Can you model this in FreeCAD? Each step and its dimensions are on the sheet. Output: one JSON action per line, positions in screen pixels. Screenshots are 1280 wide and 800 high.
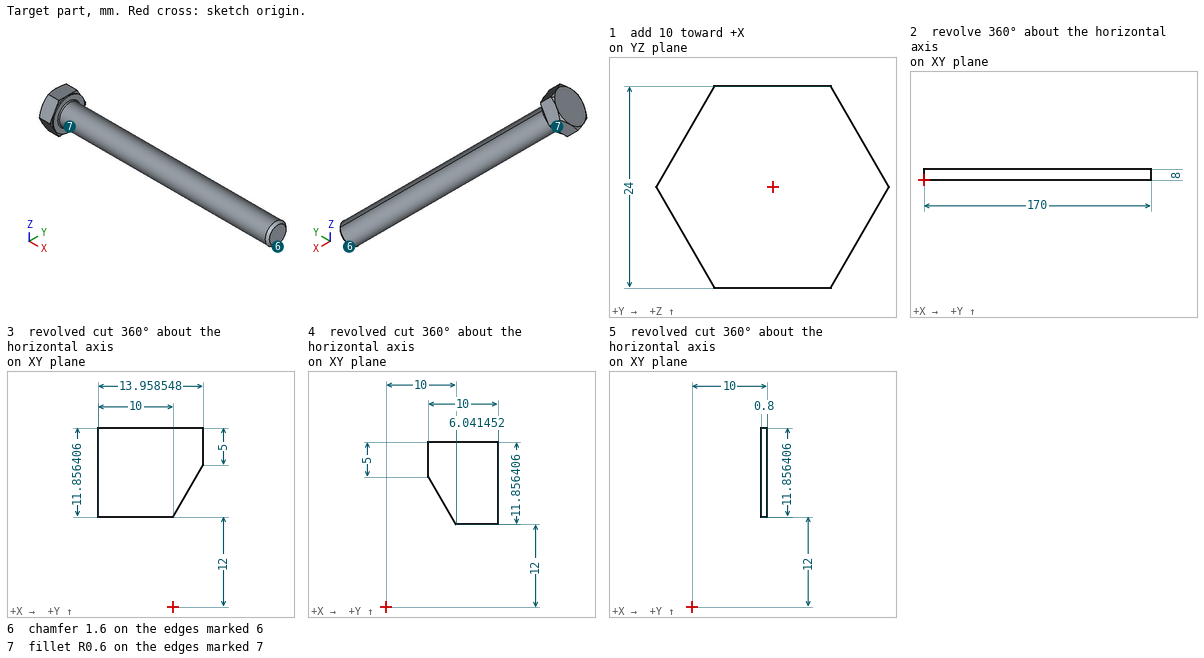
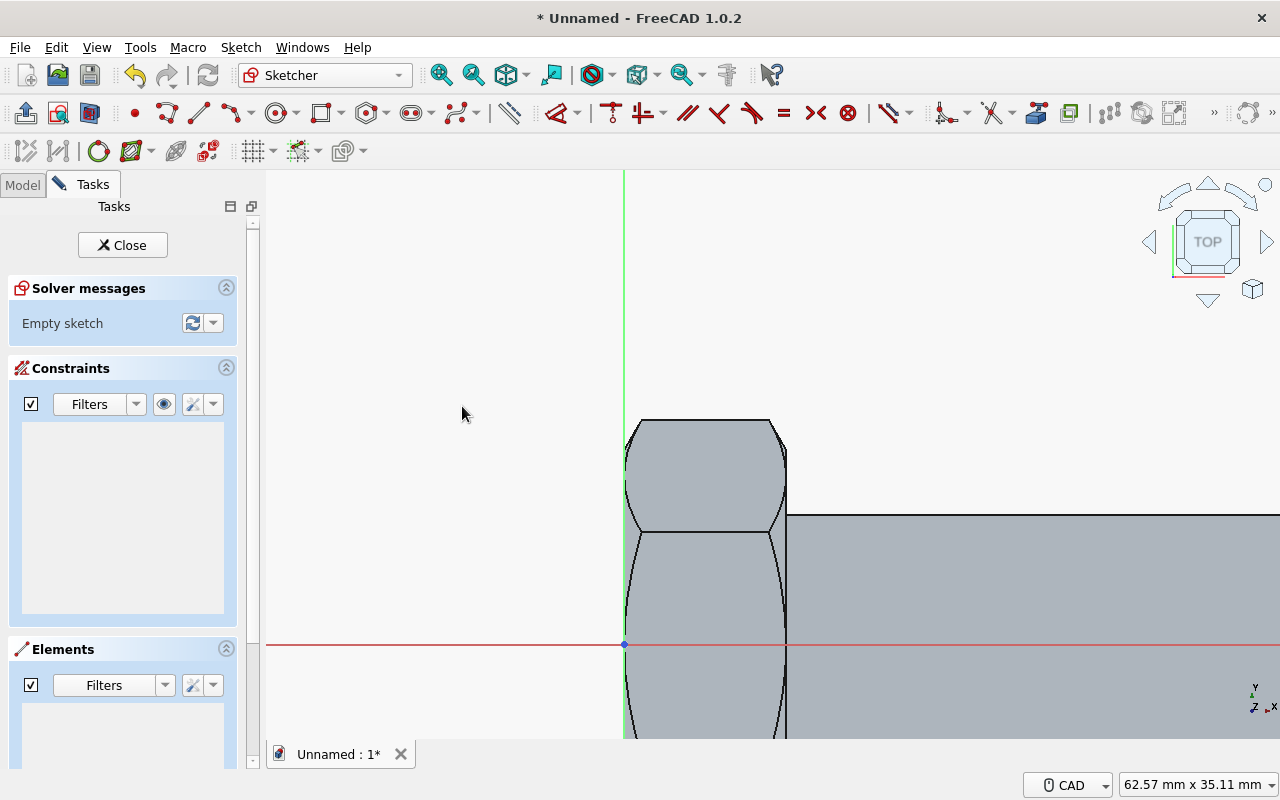
{"action": "left_click", "coordinate": [322, 114]}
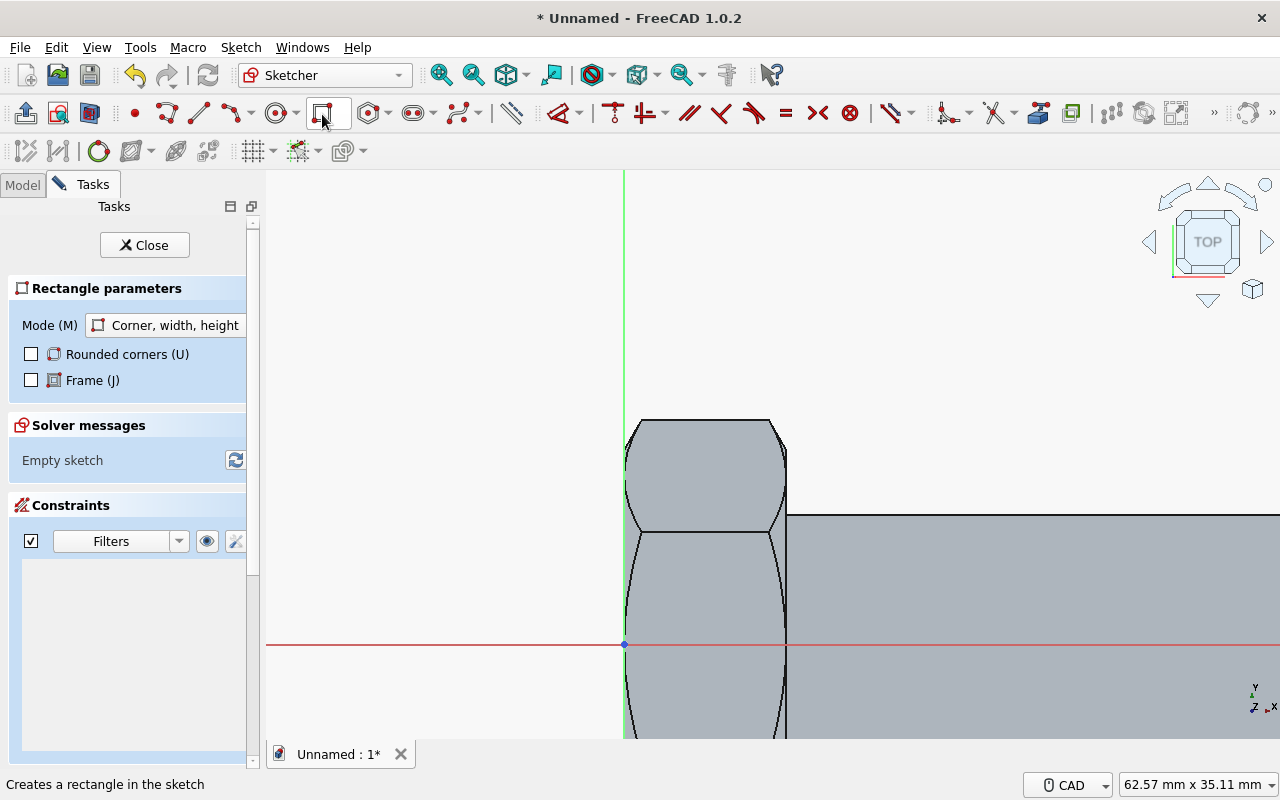
{"action": "scroll", "coordinate": [773, 258], "scroll_direction": "up", "scroll_amount": 2}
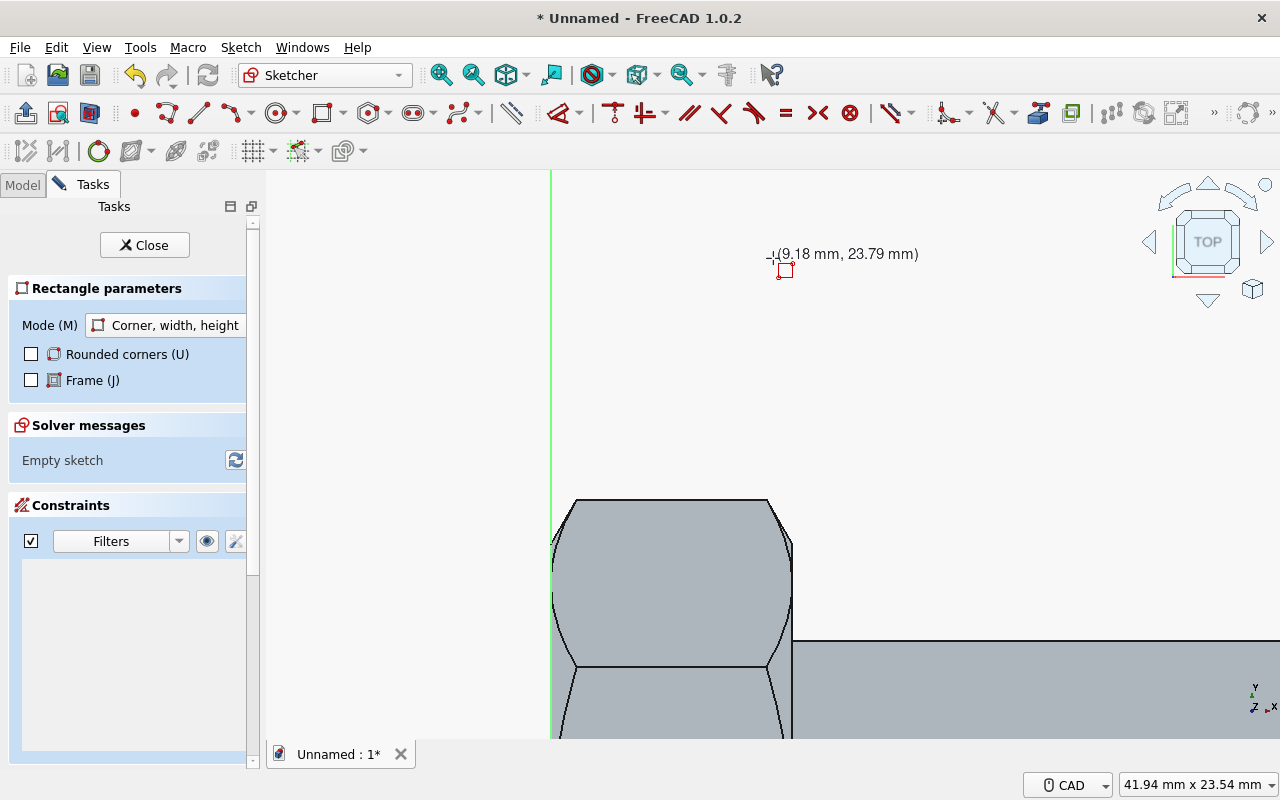
{"action": "left_click", "coordinate": [773, 258]}
{"action": "left_click", "coordinate": [792, 545]}
{"action": "key", "text": "Escape"}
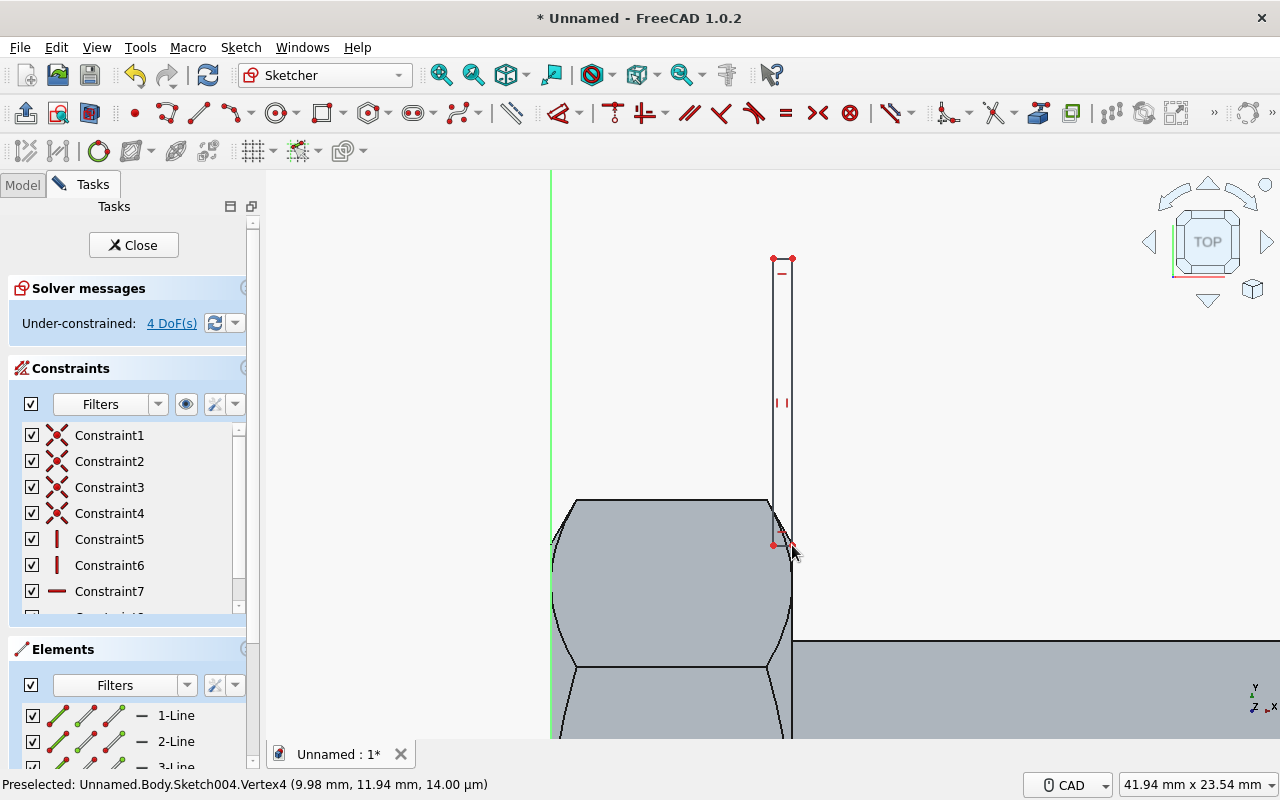
{"action": "left_click", "coordinate": [558, 114]}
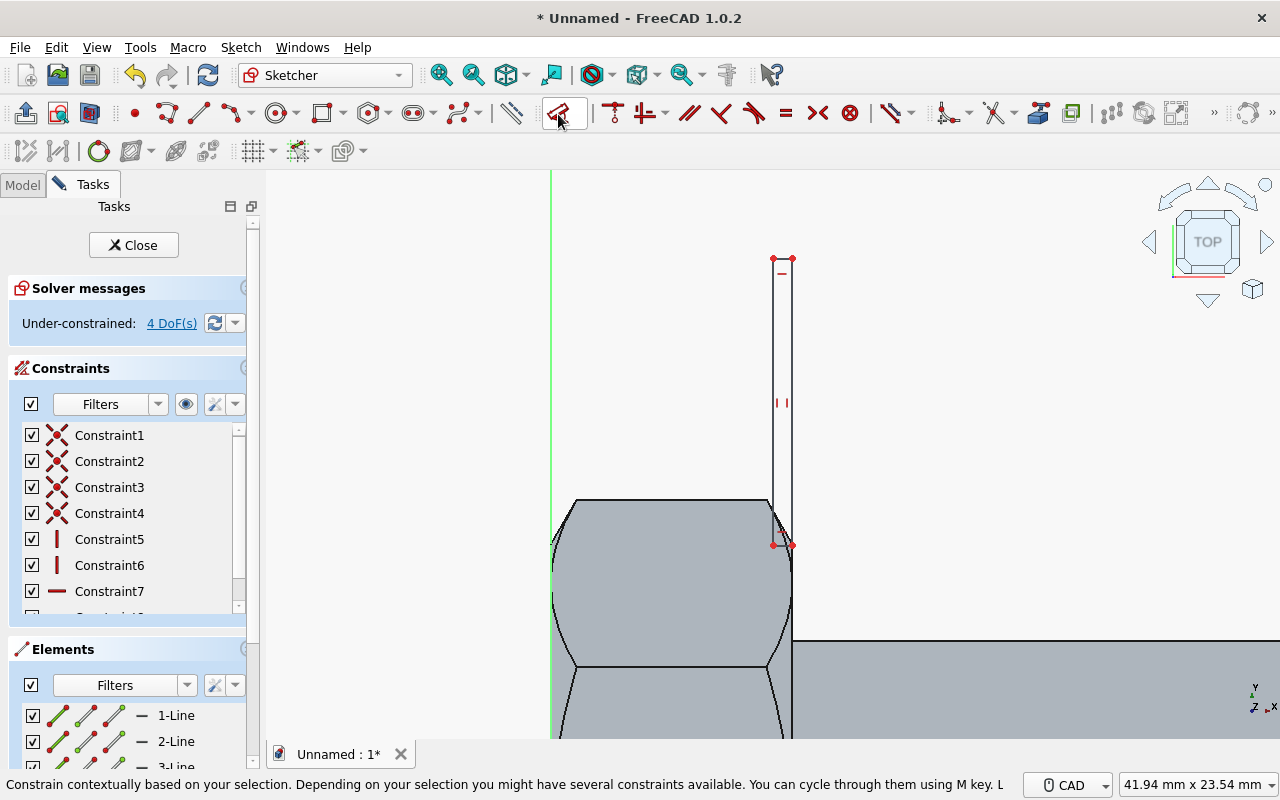
{"action": "scroll", "coordinate": [782, 546], "scroll_direction": "up", "scroll_amount": 4}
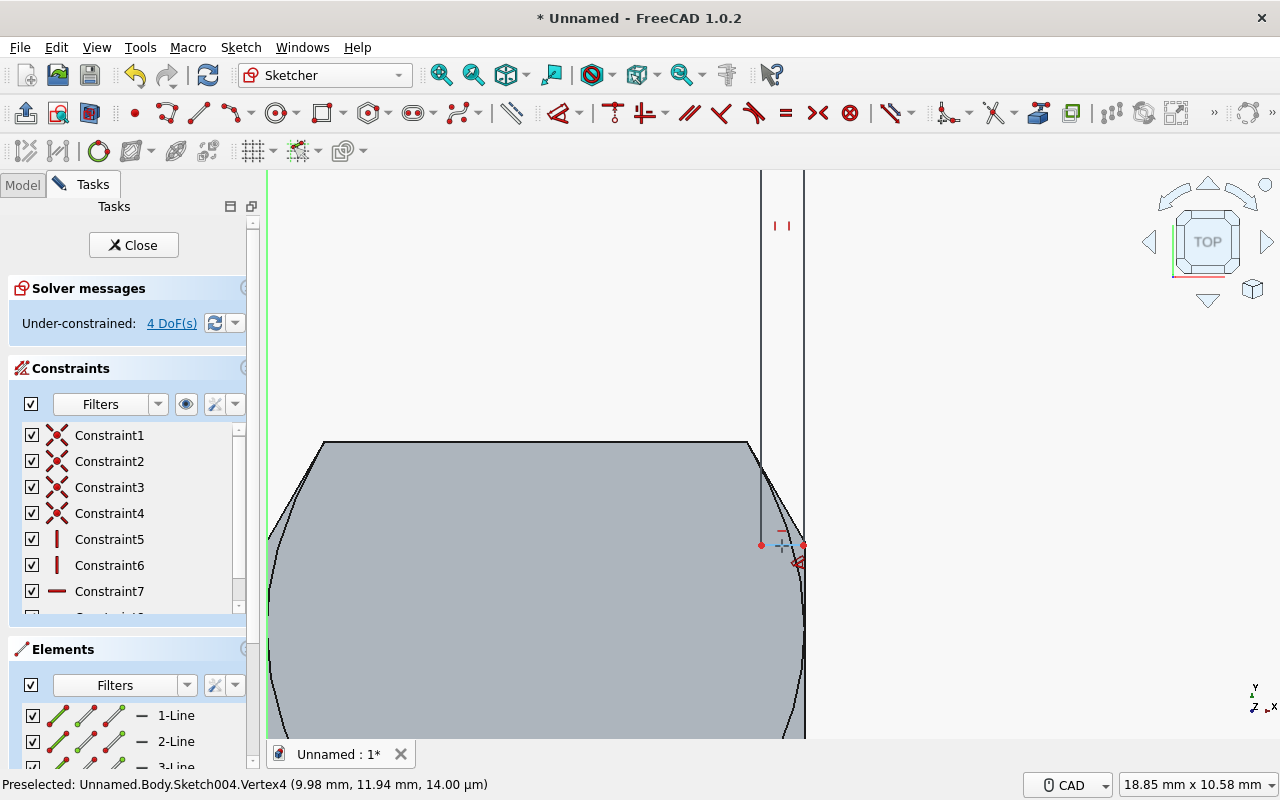
{"action": "left_click", "coordinate": [782, 545]}
{"action": "left_click", "coordinate": [782, 511]}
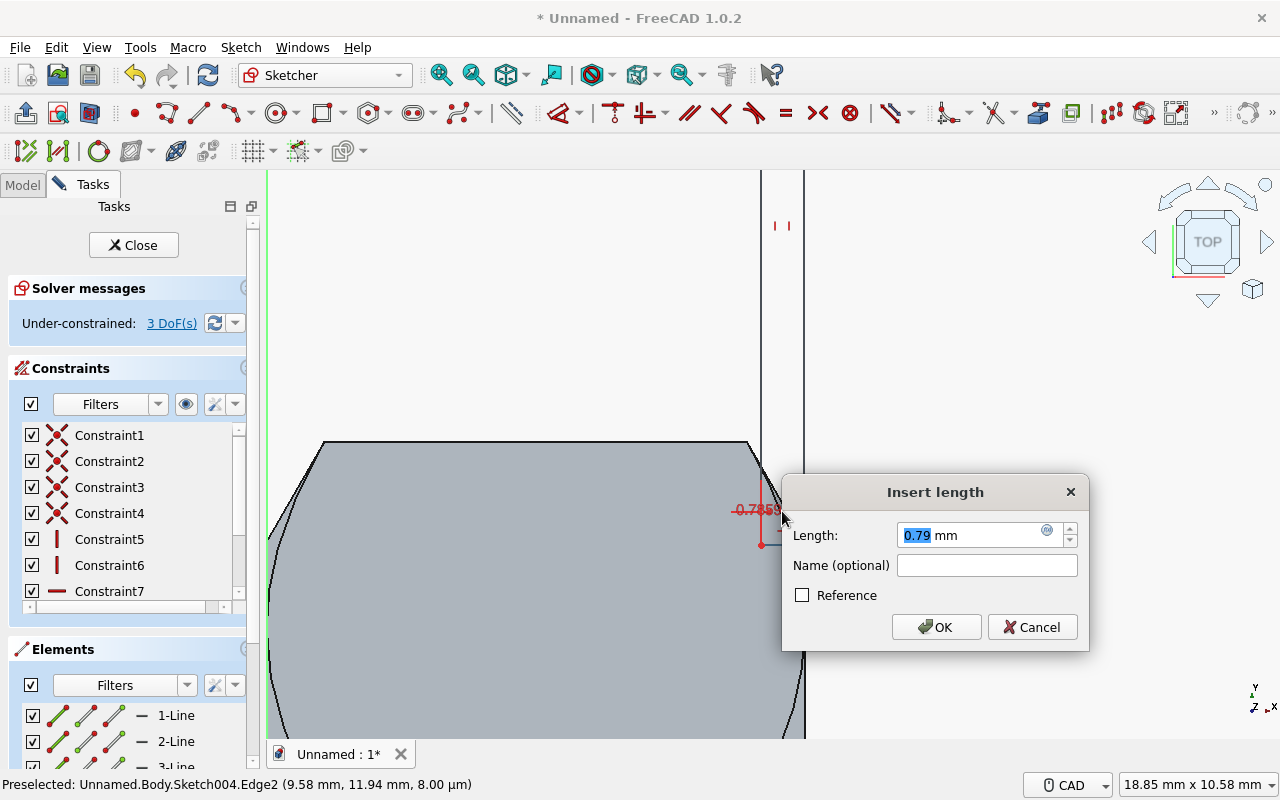
{"action": "type", "text": "0.8"}
{"action": "key", "text": "Return"}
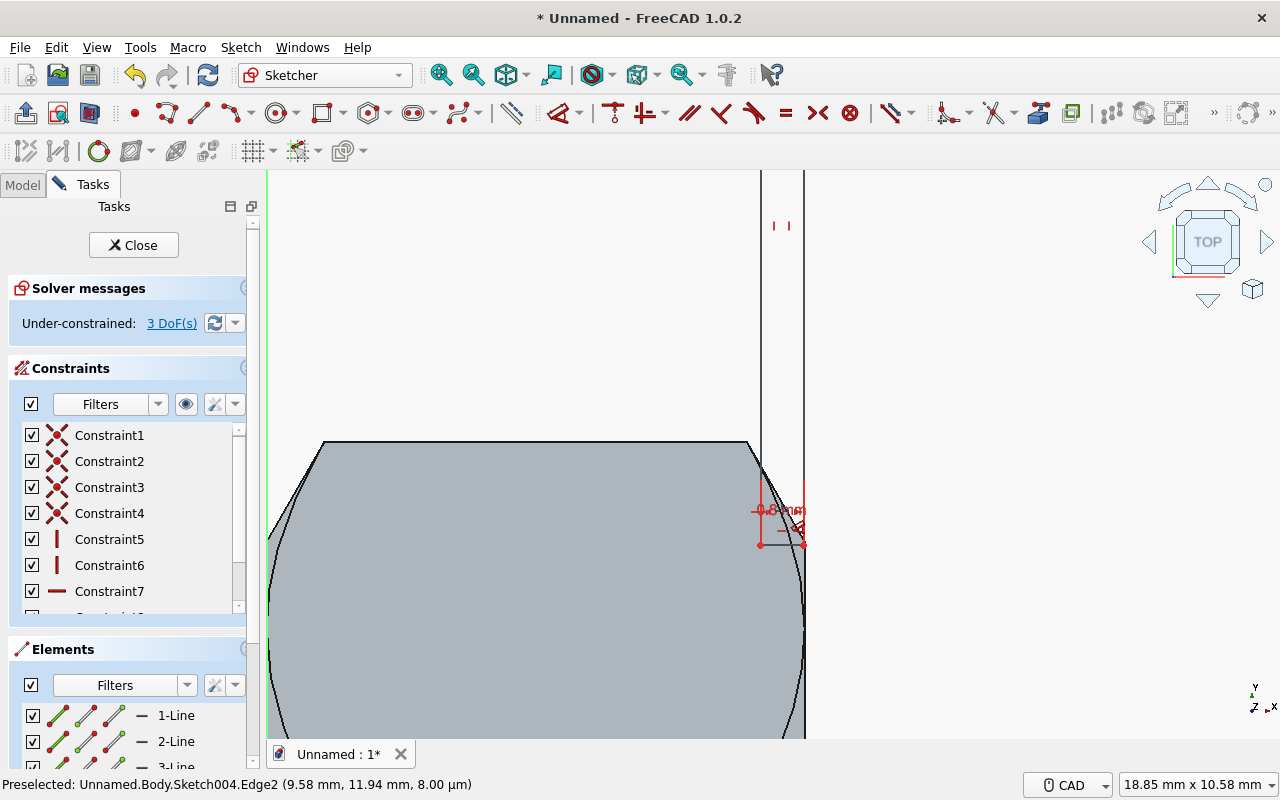
{"action": "left_click", "coordinate": [761, 545]}
{"action": "left_click", "coordinate": [795, 628]}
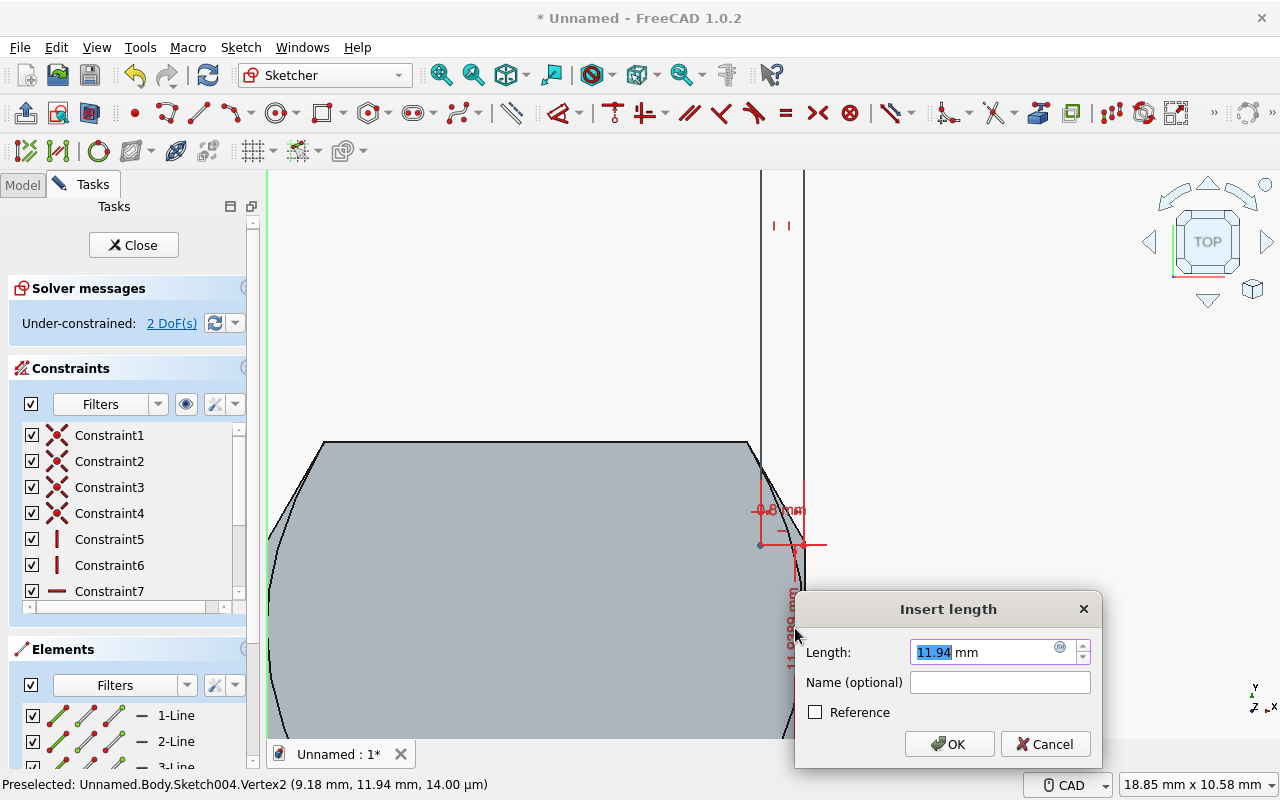
{"action": "type", "text": "12"}
{"action": "key", "text": "Return"}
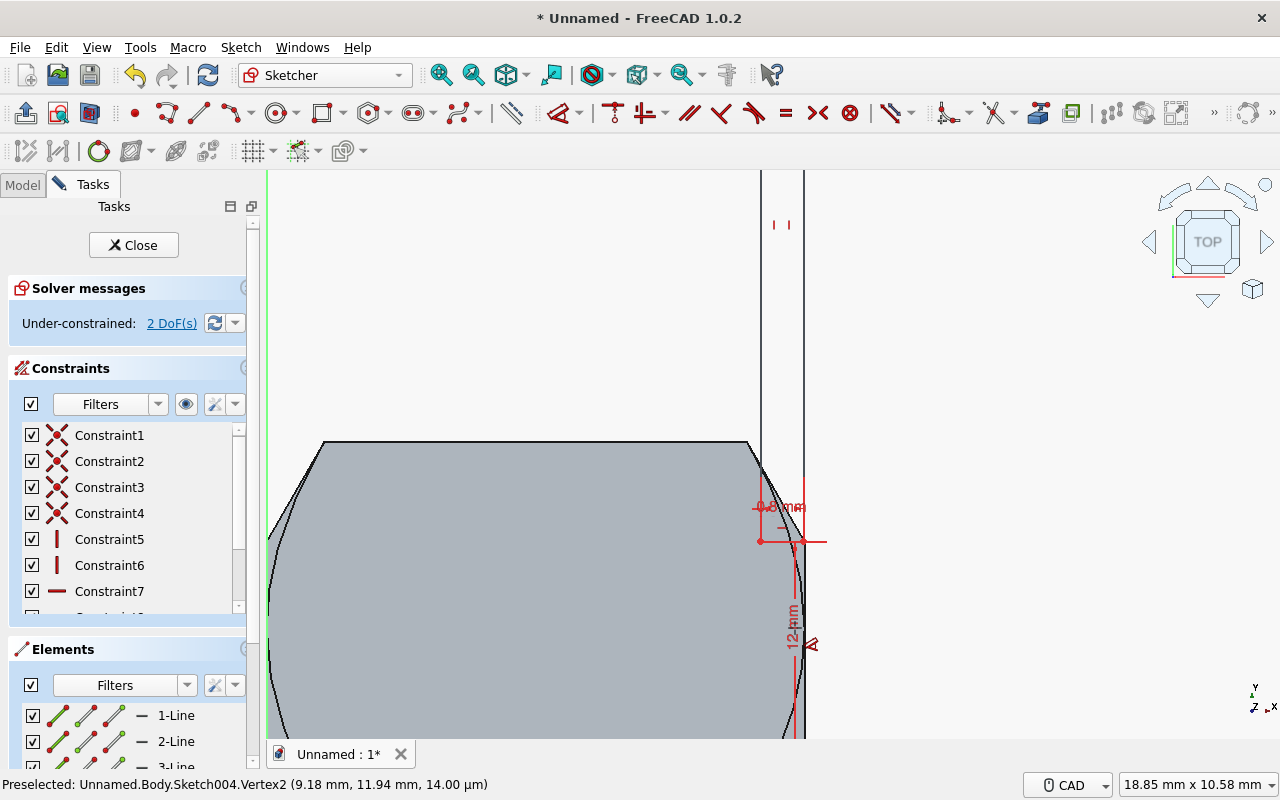
{"action": "left_click", "coordinate": [804, 542]}
{"action": "left_click", "coordinate": [549, 508]}